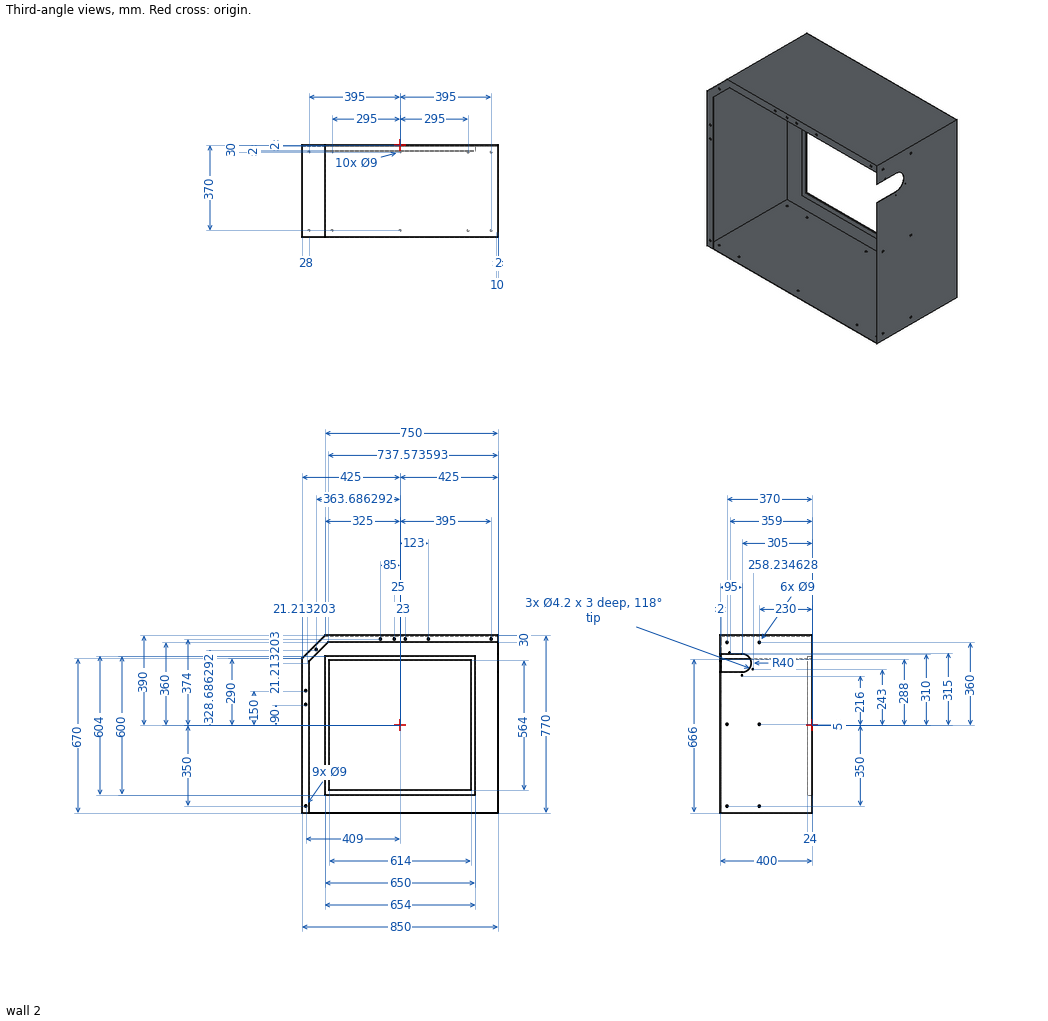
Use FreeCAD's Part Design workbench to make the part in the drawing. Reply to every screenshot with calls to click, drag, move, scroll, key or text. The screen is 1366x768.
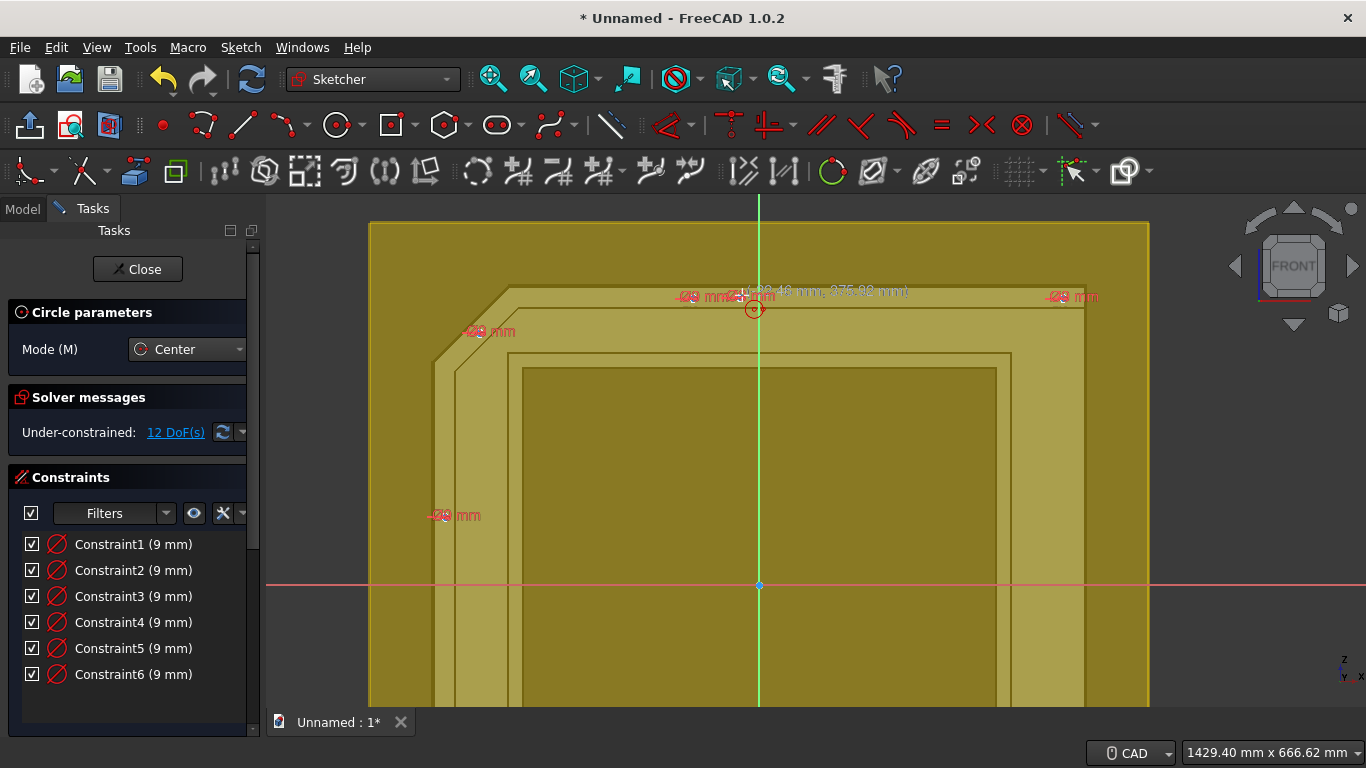
scroll(445, 470, up, 10)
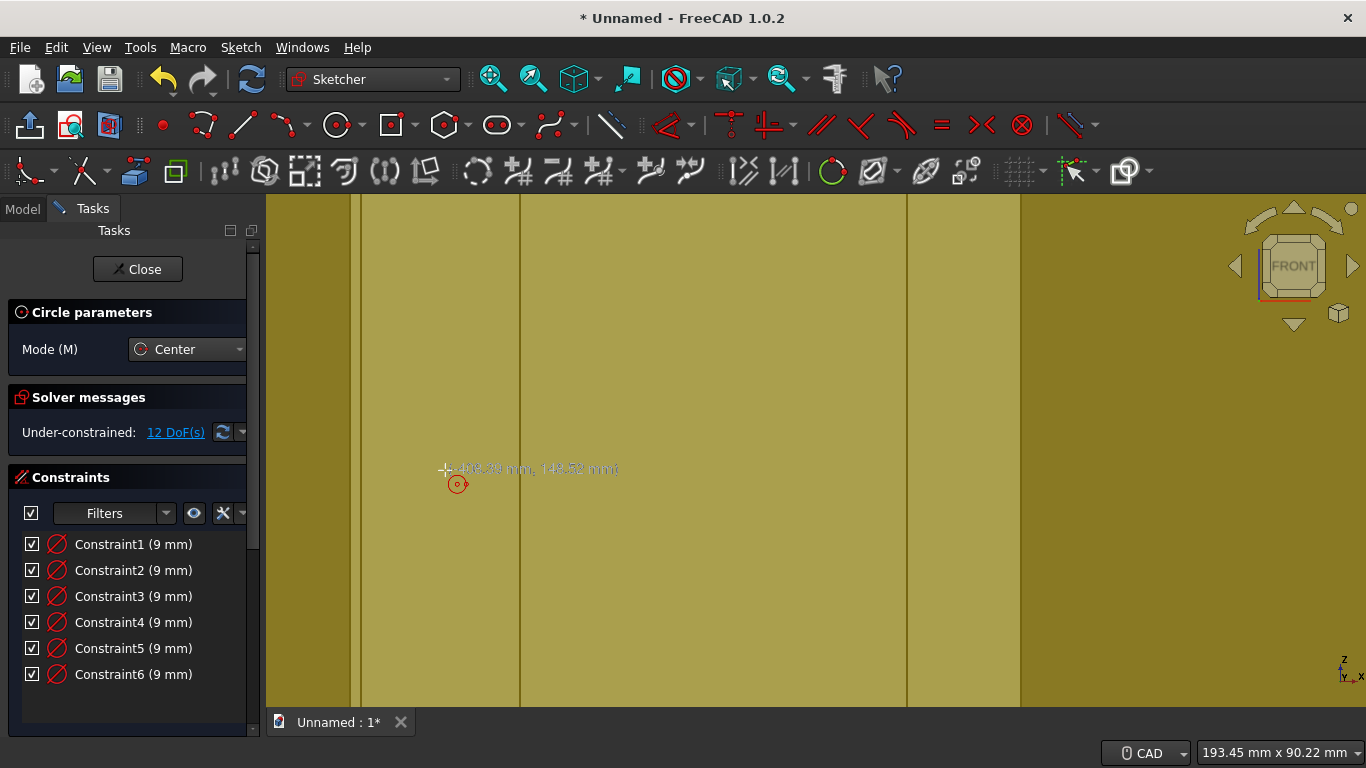
scroll(589, 386, down, 13)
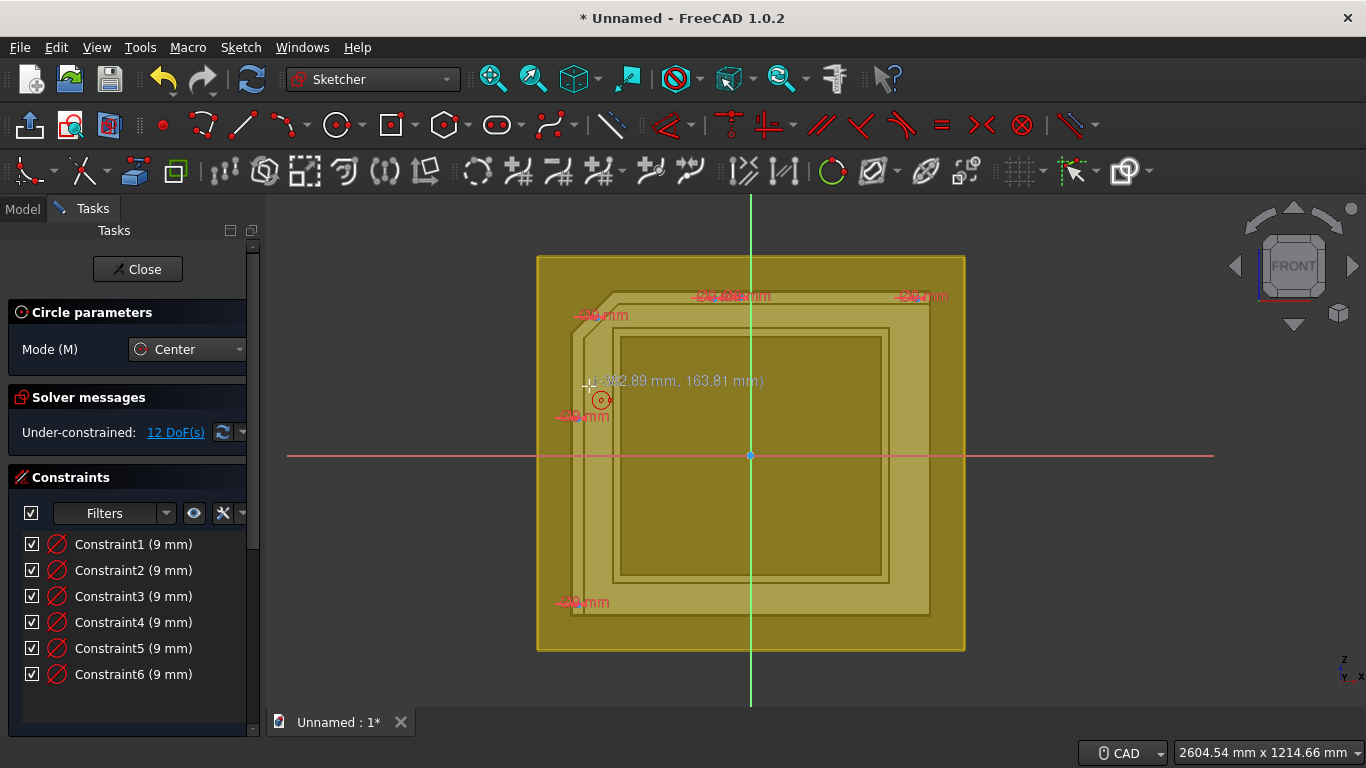
click(578, 392)
move(580, 391)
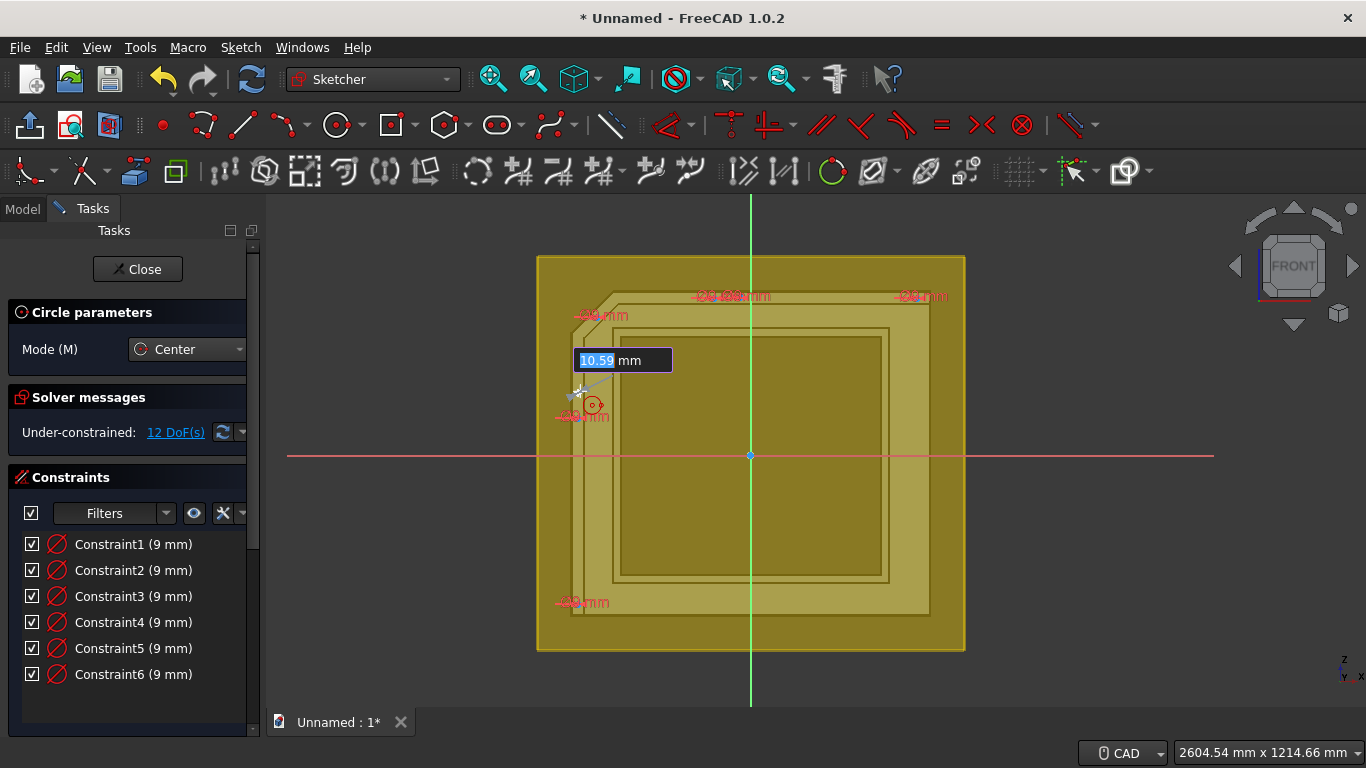
text(9)
key(Return)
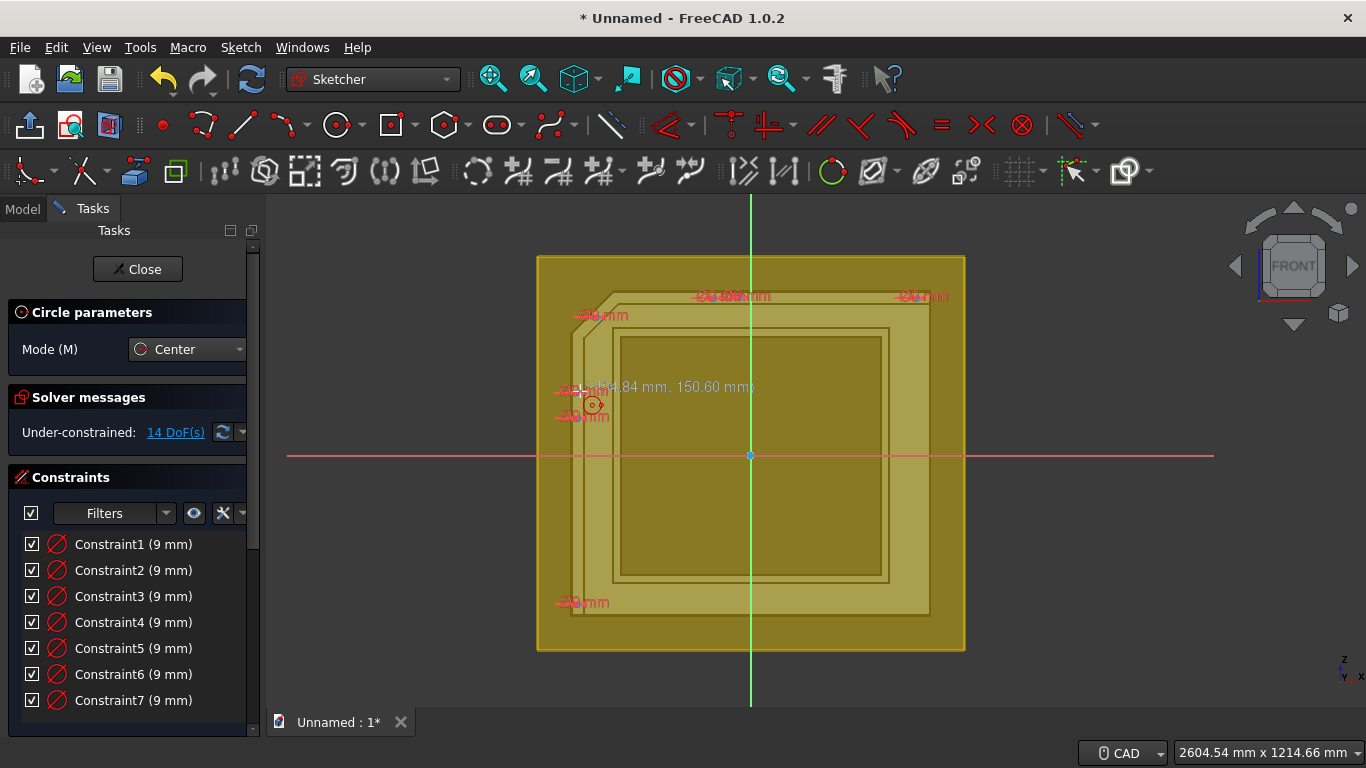
scroll(761, 298, up, 13)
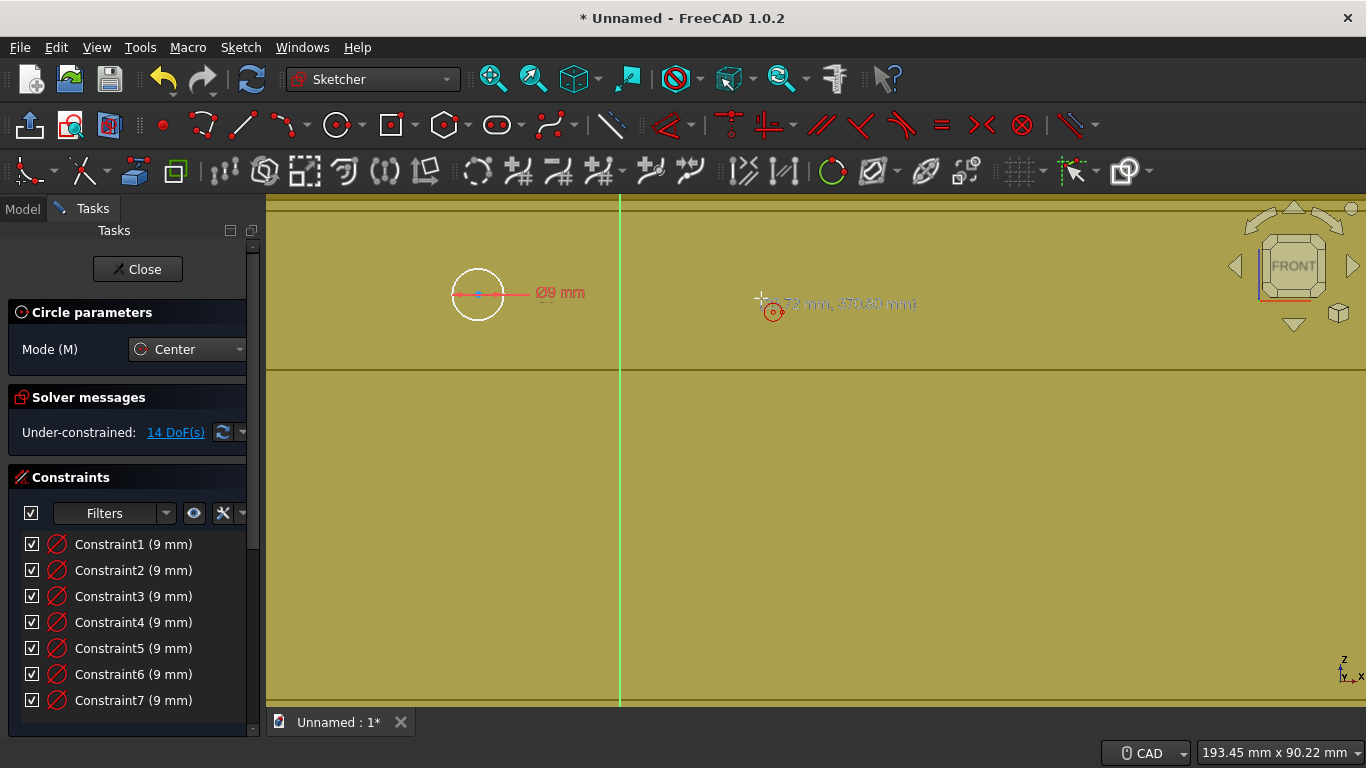
scroll(761, 298, down, 13)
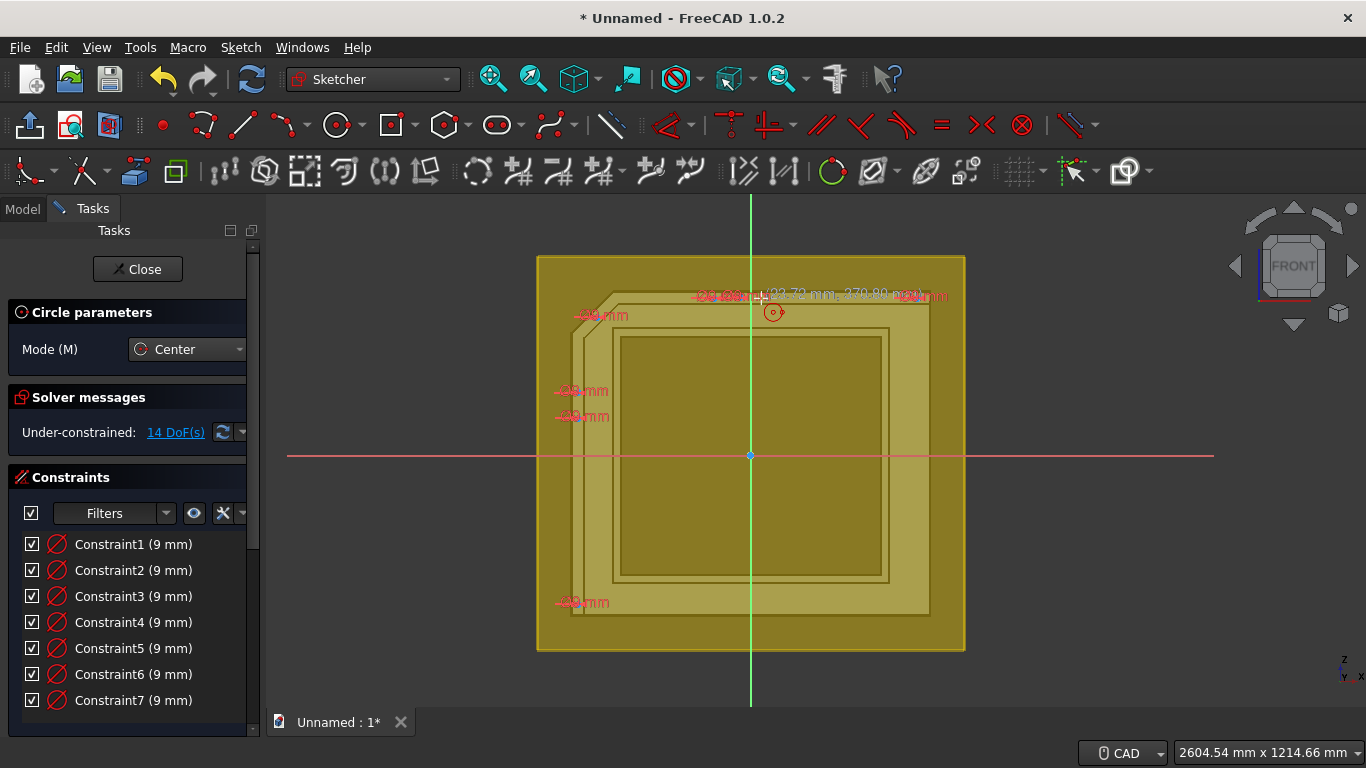
scroll(761, 298, up, 3)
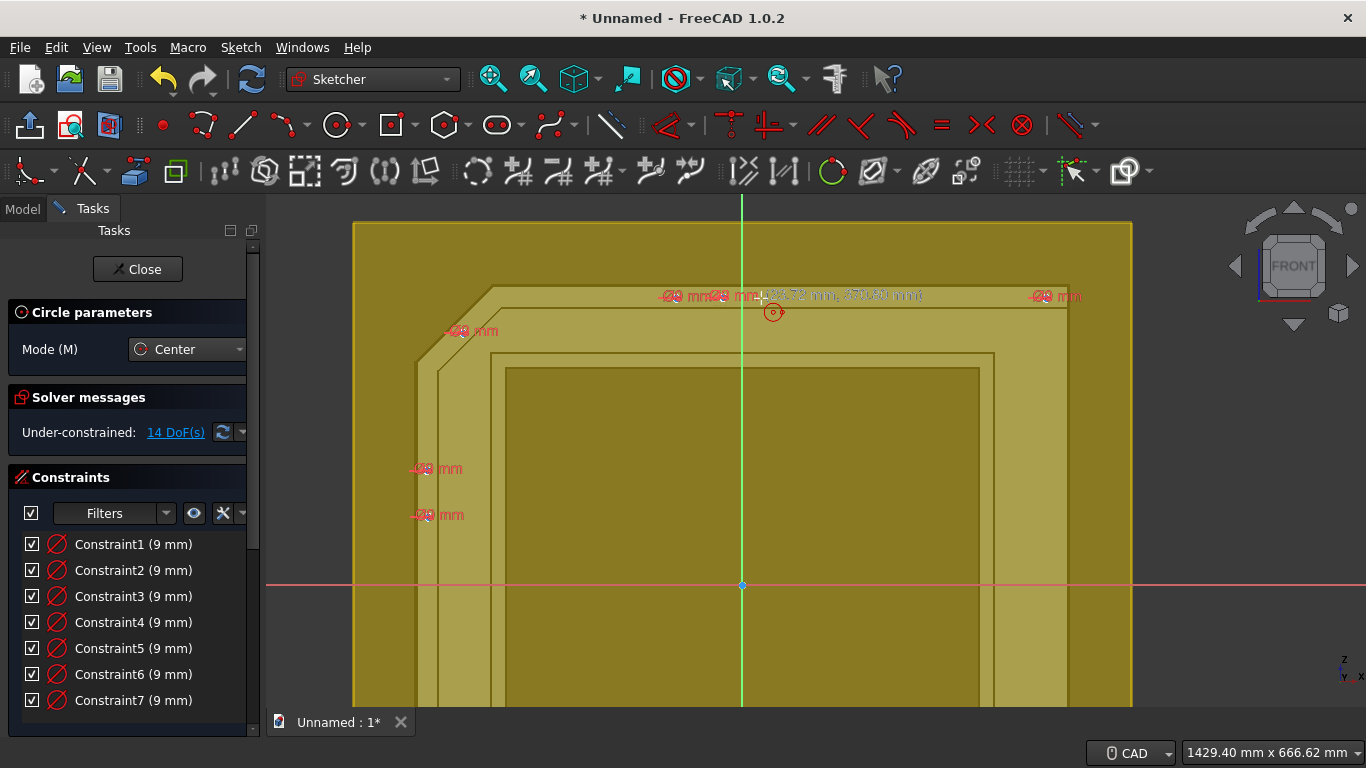
click(760, 297)
move(763, 295)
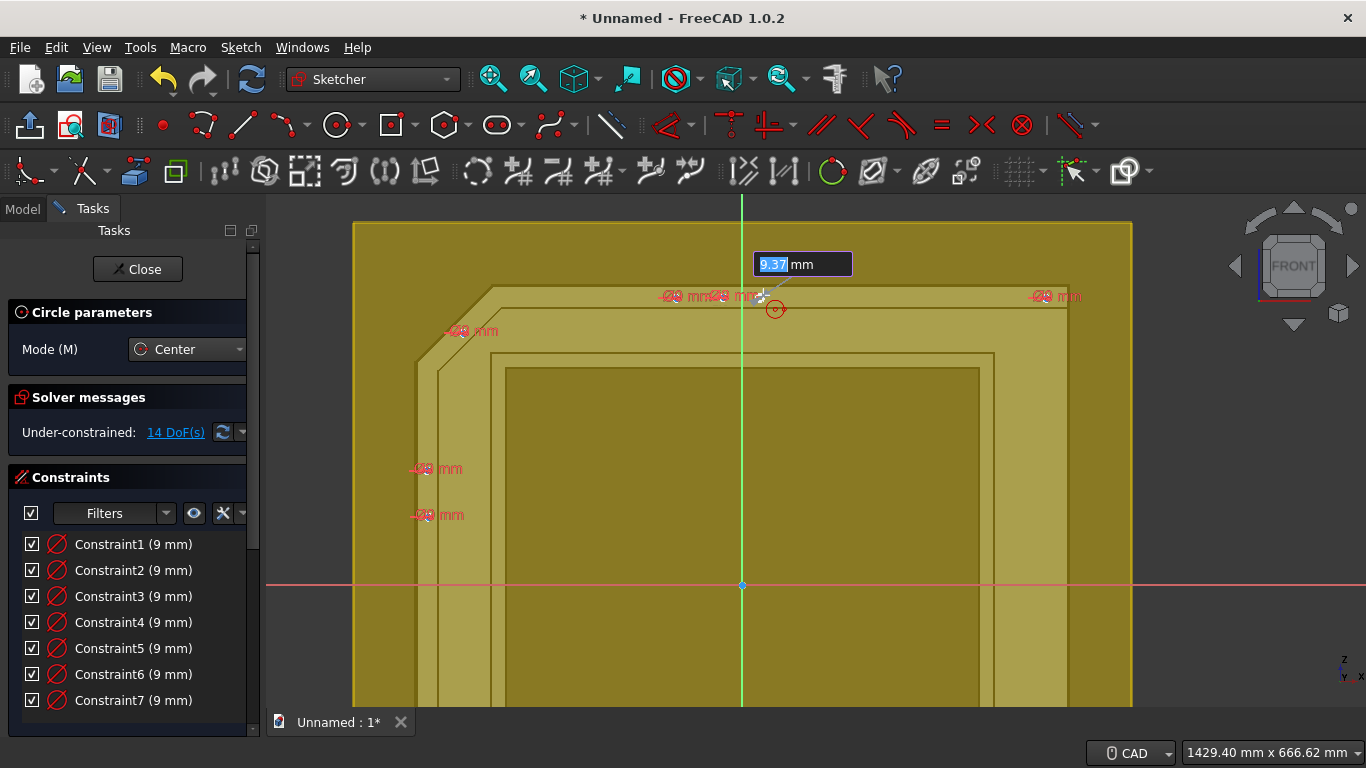
text(9)
key(Return)